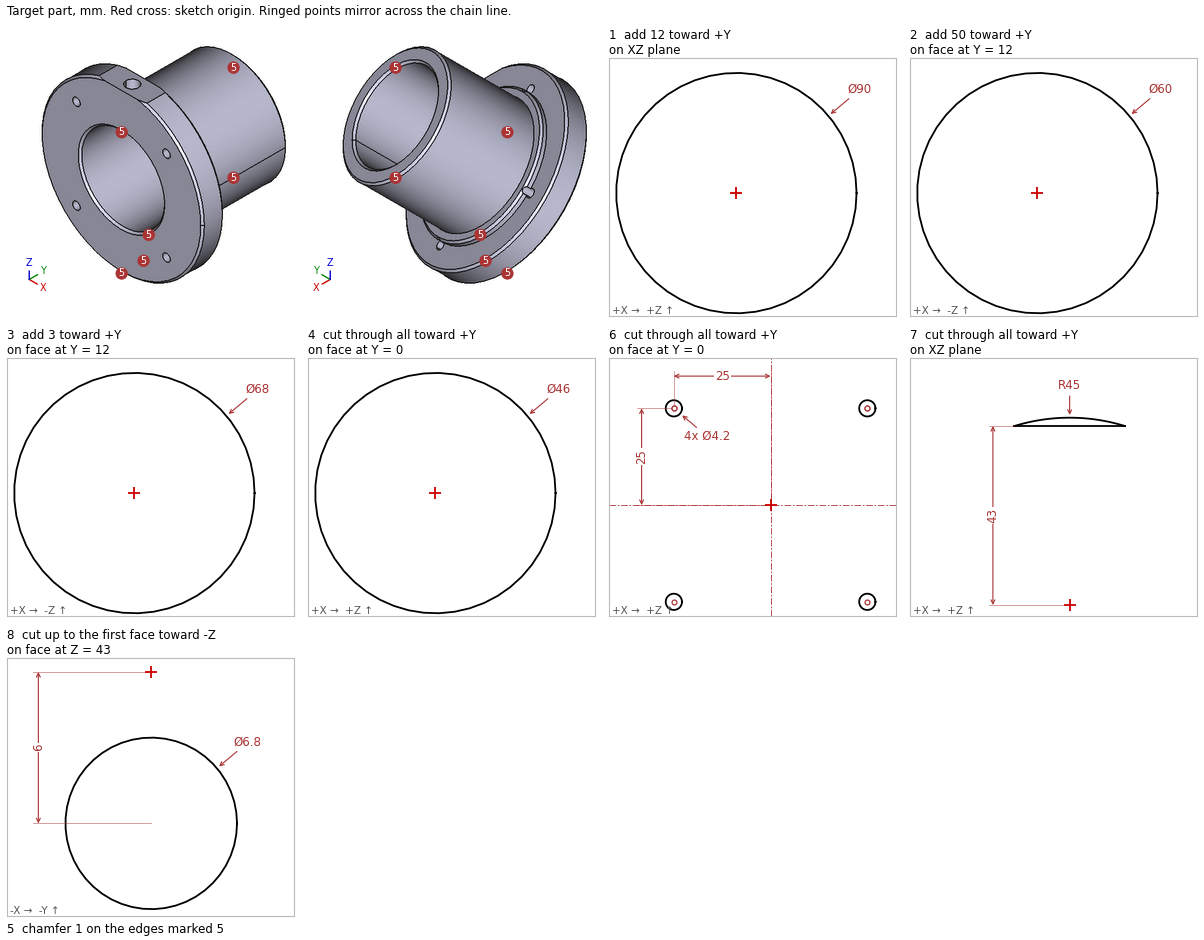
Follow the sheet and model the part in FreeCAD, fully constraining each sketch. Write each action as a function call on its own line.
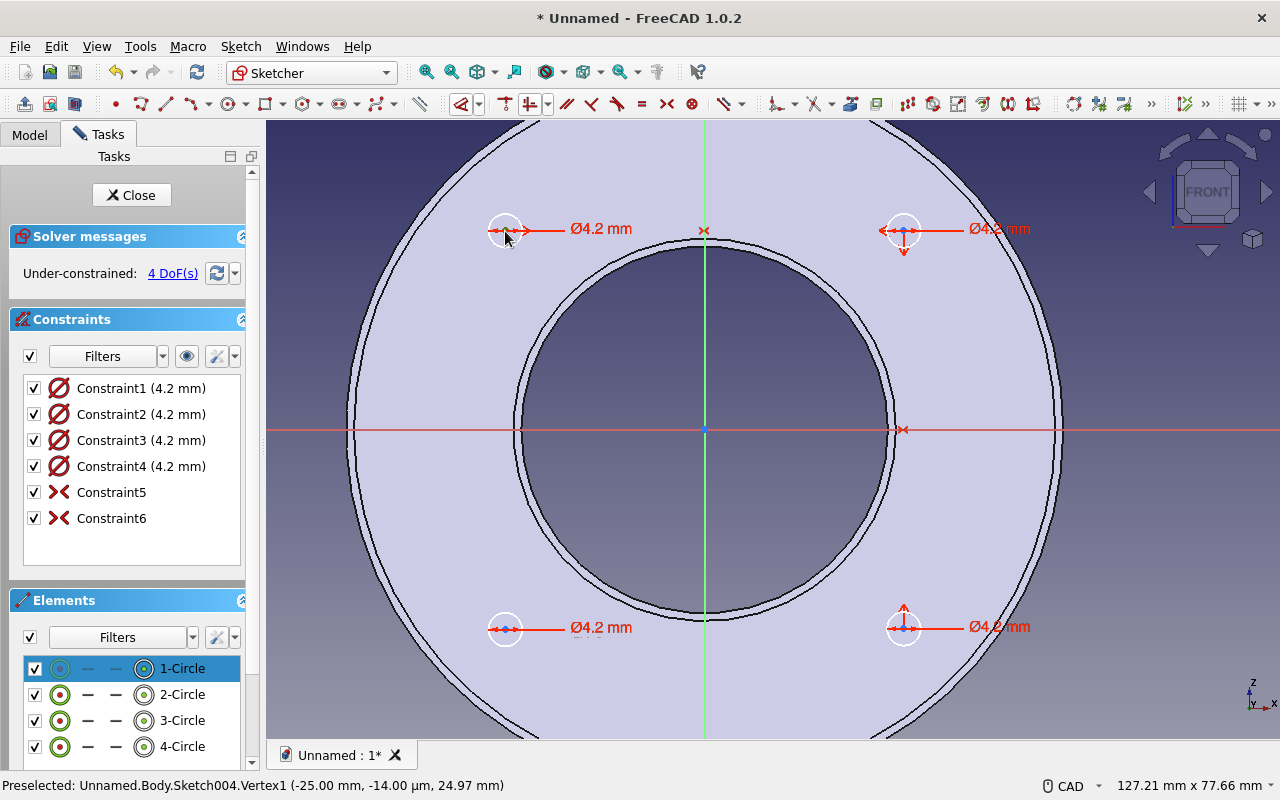
click(505, 630)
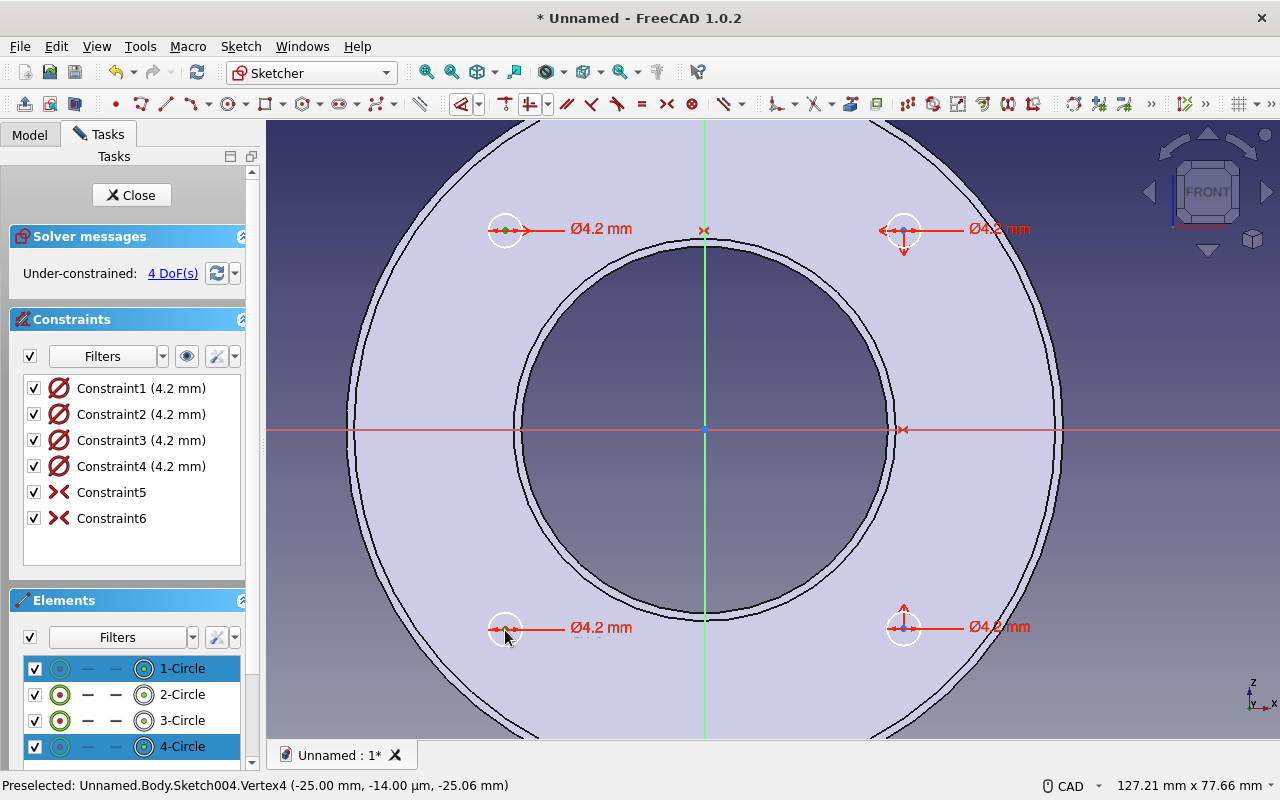
click(353, 430)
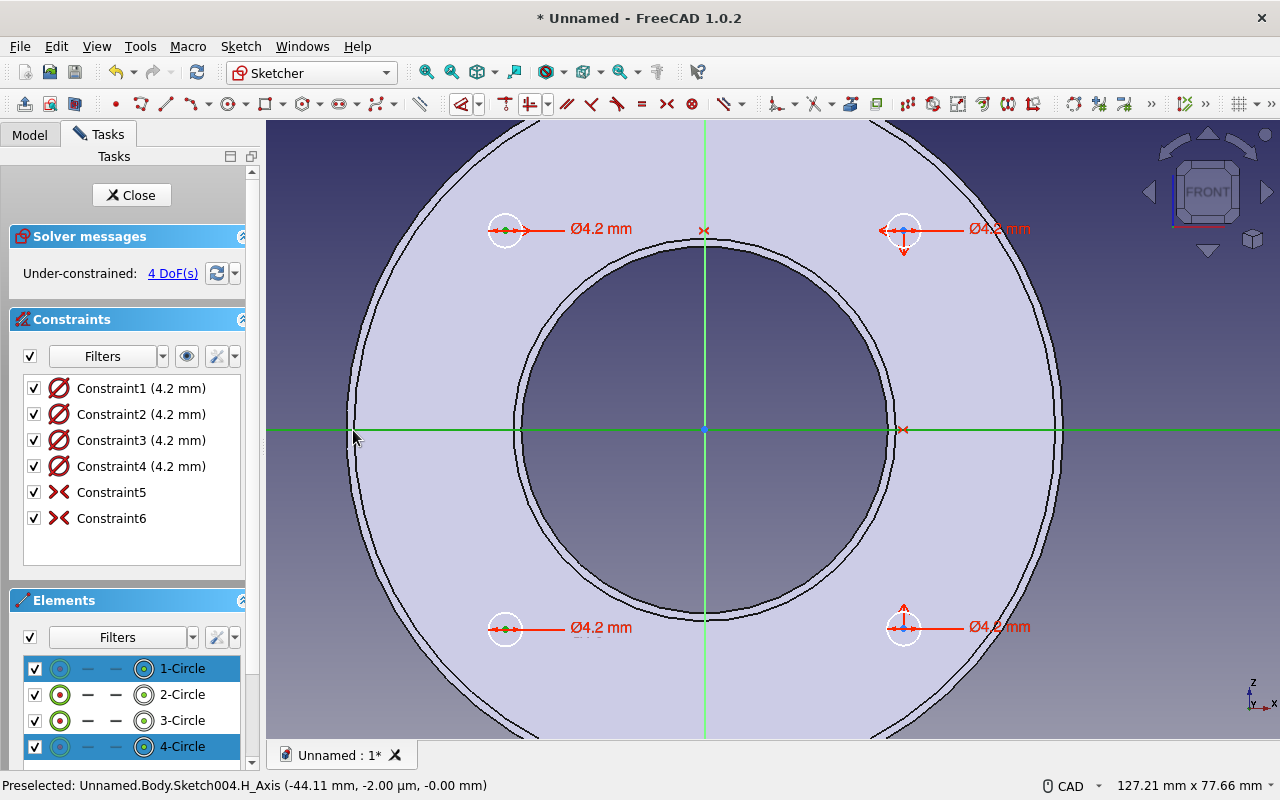
click(667, 104)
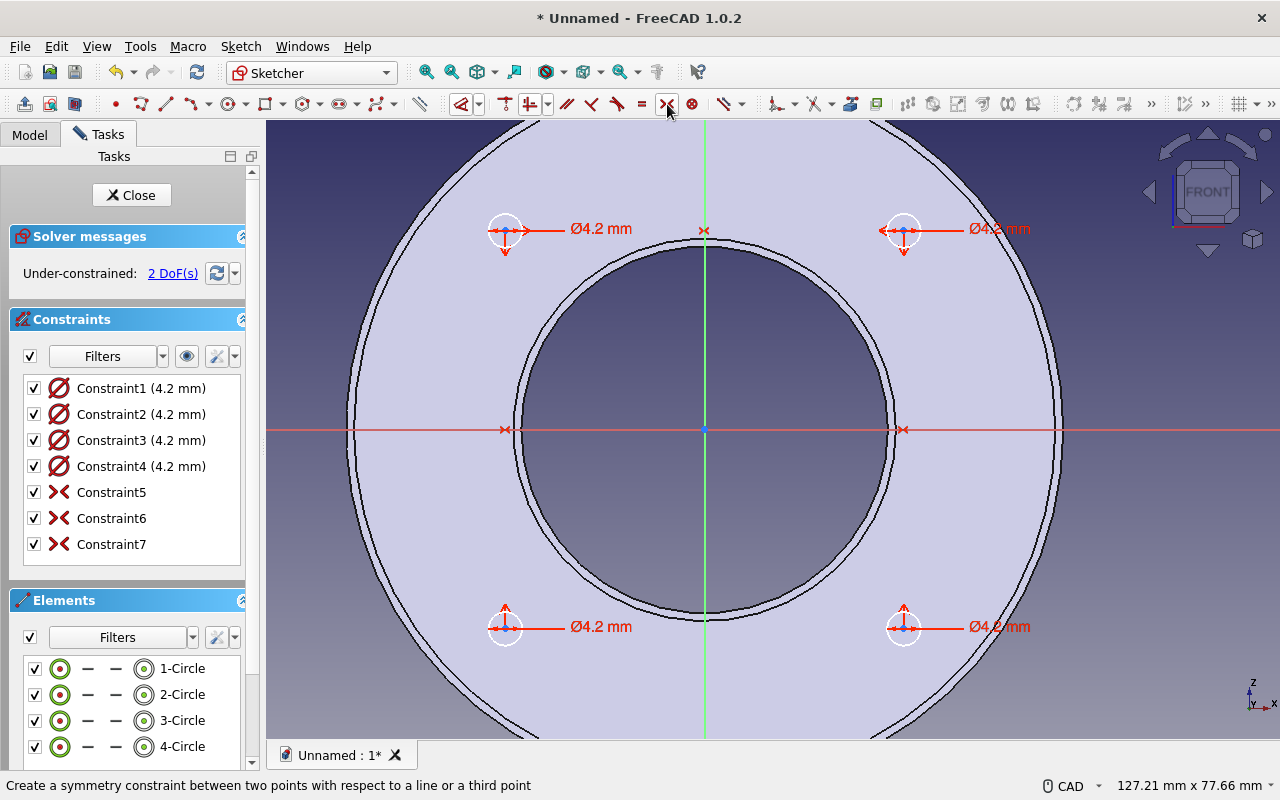
click(505, 231)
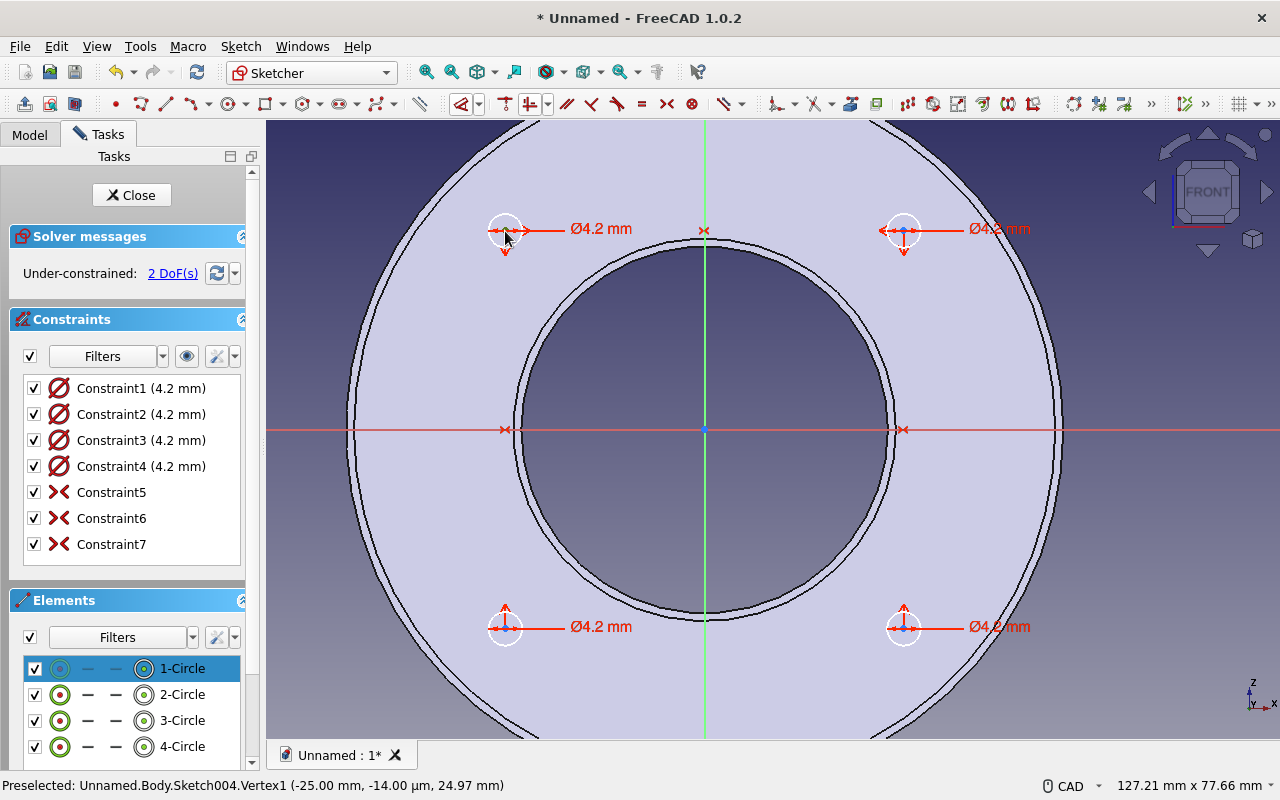
click(478, 104)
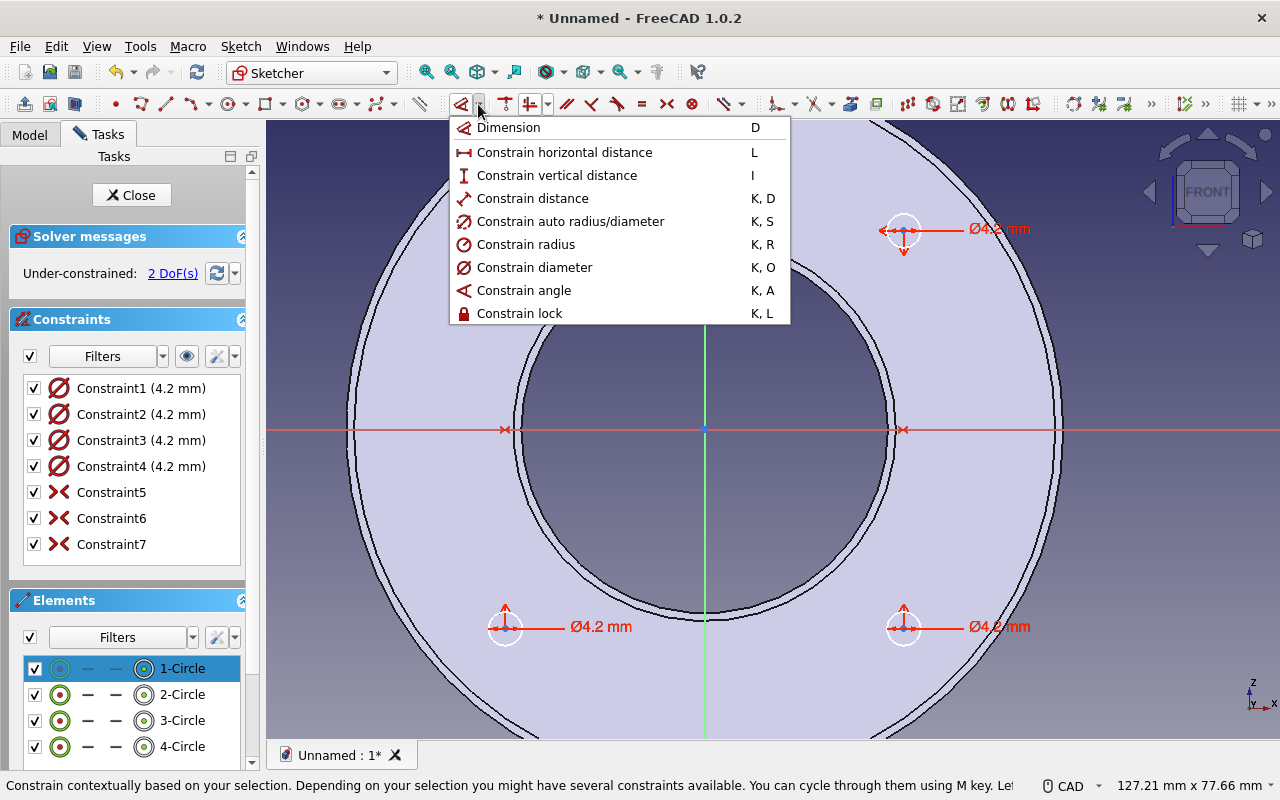
click(620, 152)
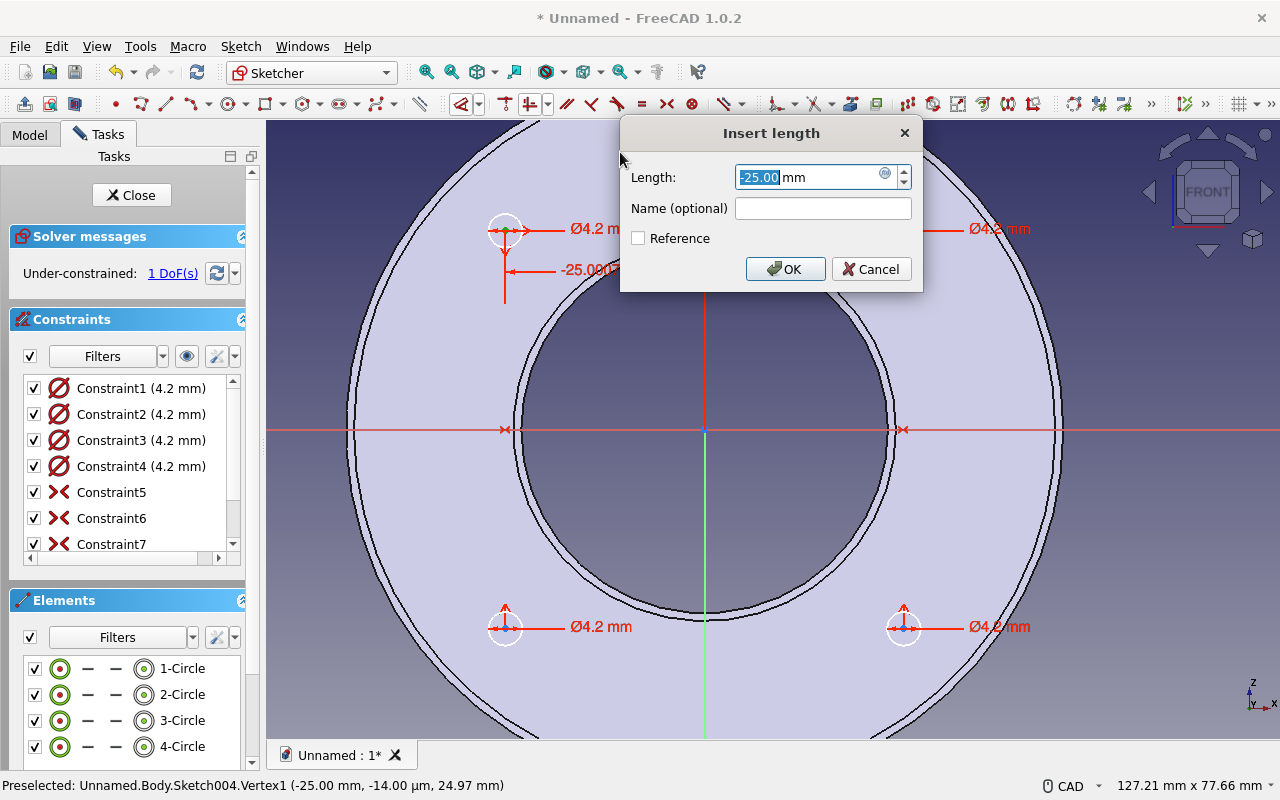
text(-25)
key(Return)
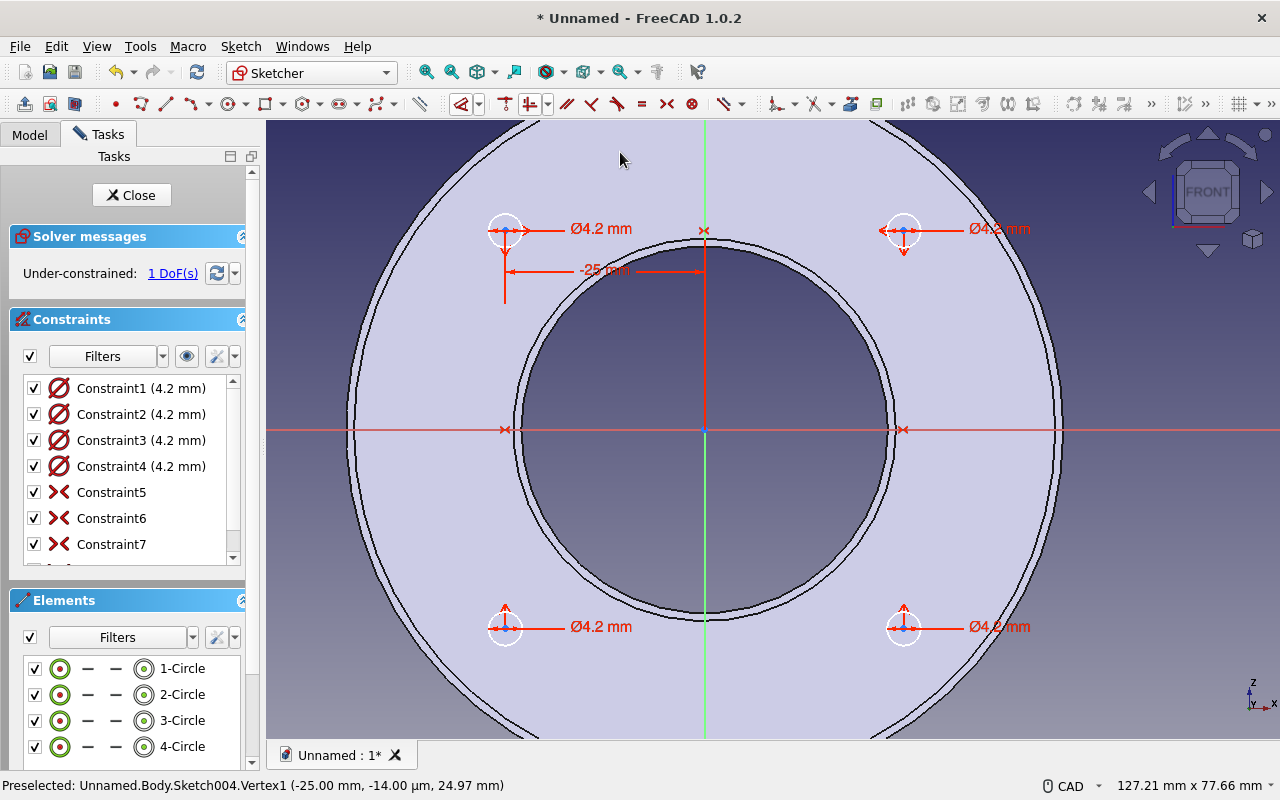
click(505, 231)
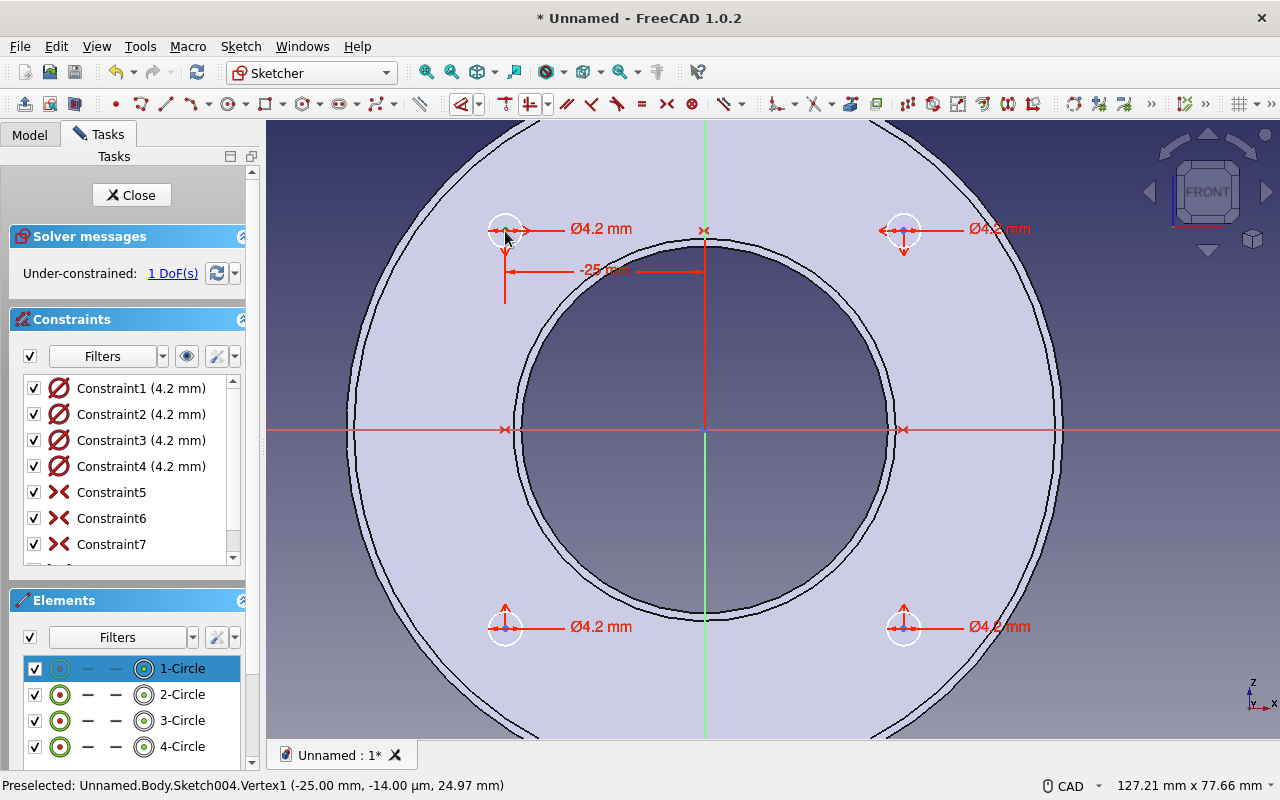
click(478, 104)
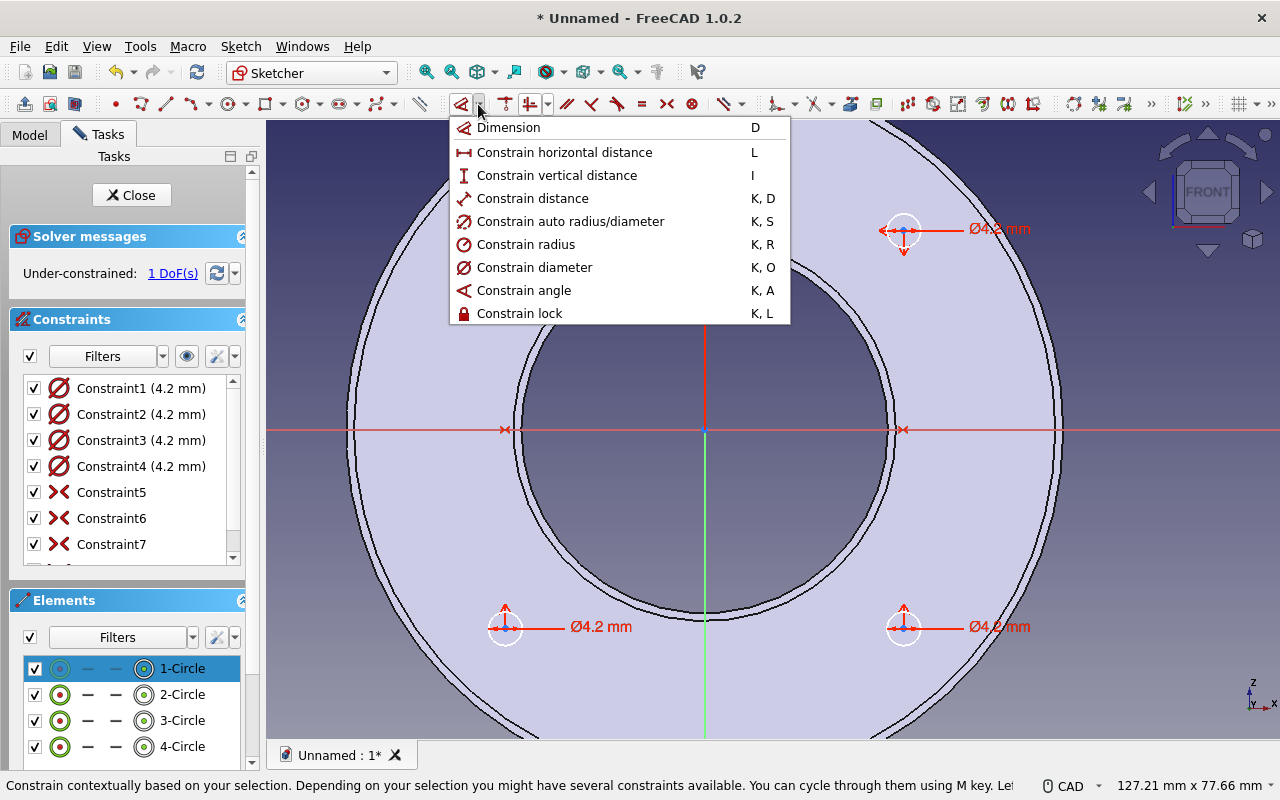
click(620, 176)